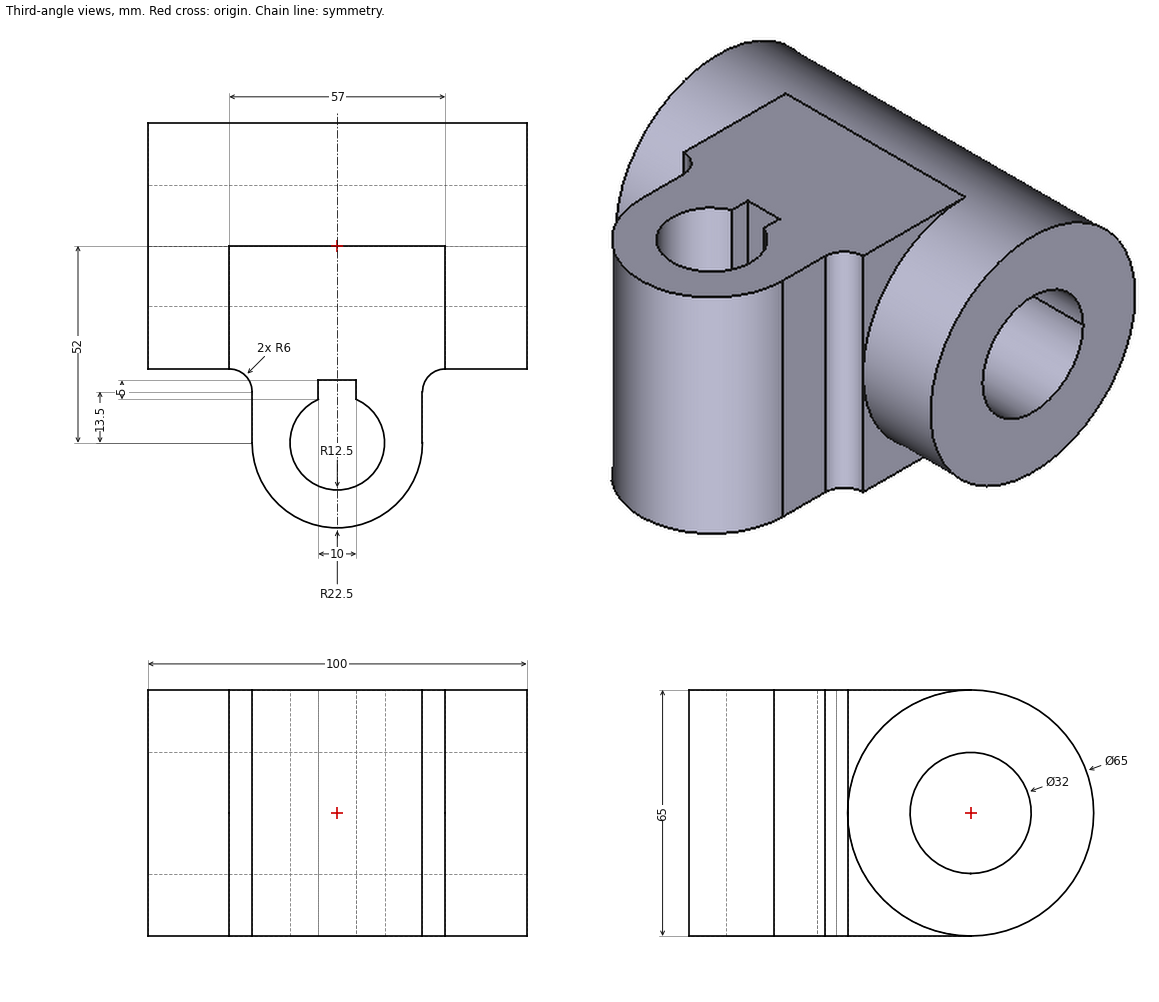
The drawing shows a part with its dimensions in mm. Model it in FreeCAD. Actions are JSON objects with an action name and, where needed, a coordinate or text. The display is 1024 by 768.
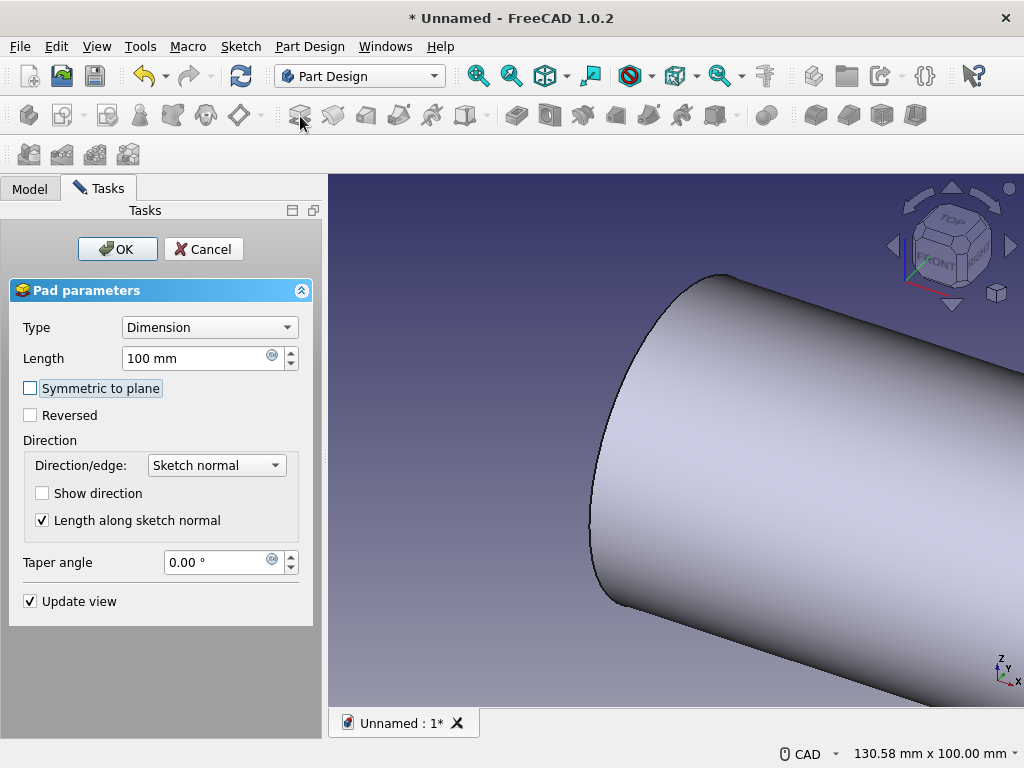
{"action": "left_click", "coordinate": [31, 388]}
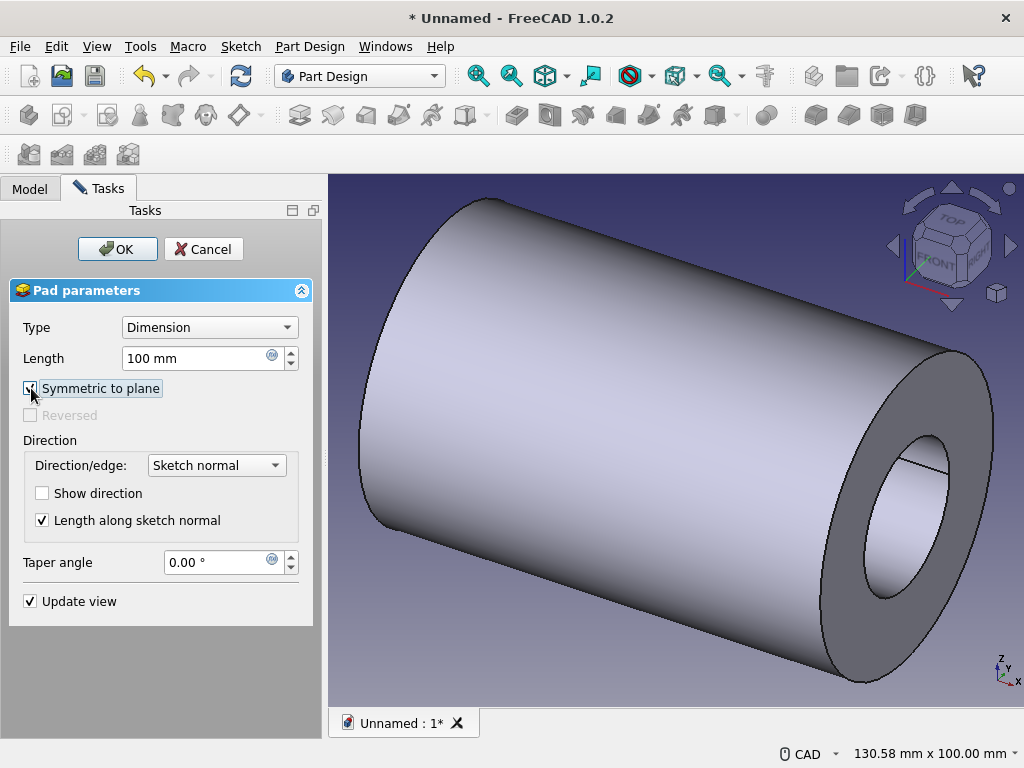
{"action": "left_click", "coordinate": [118, 249]}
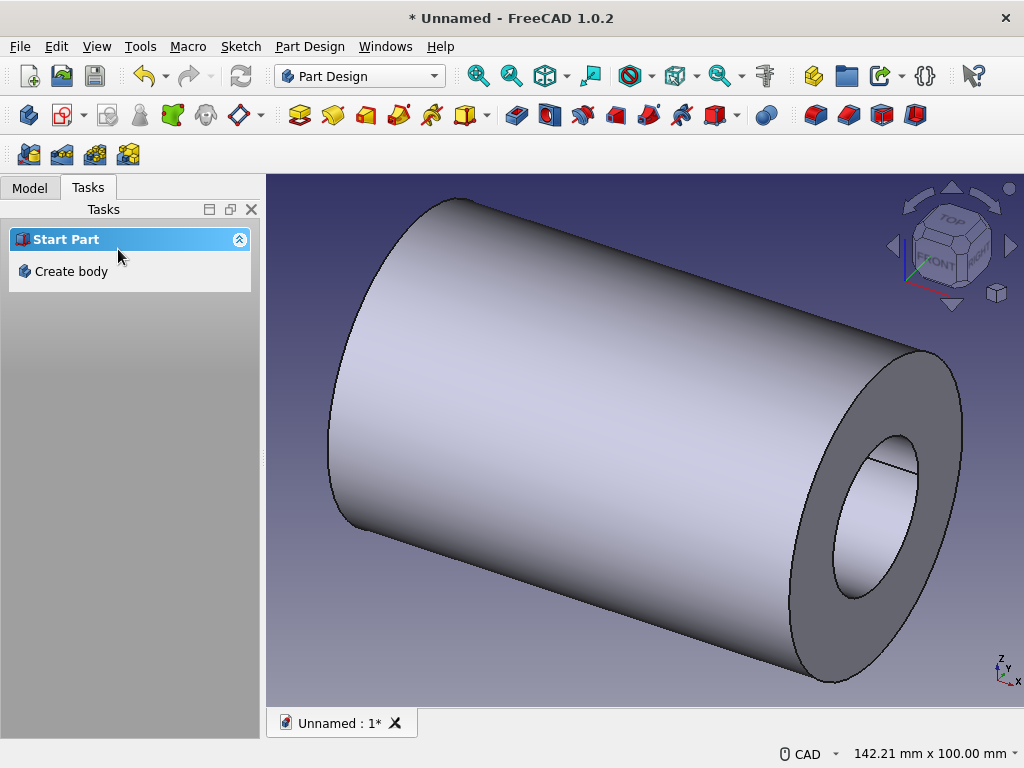
{"action": "key", "text": "v f"}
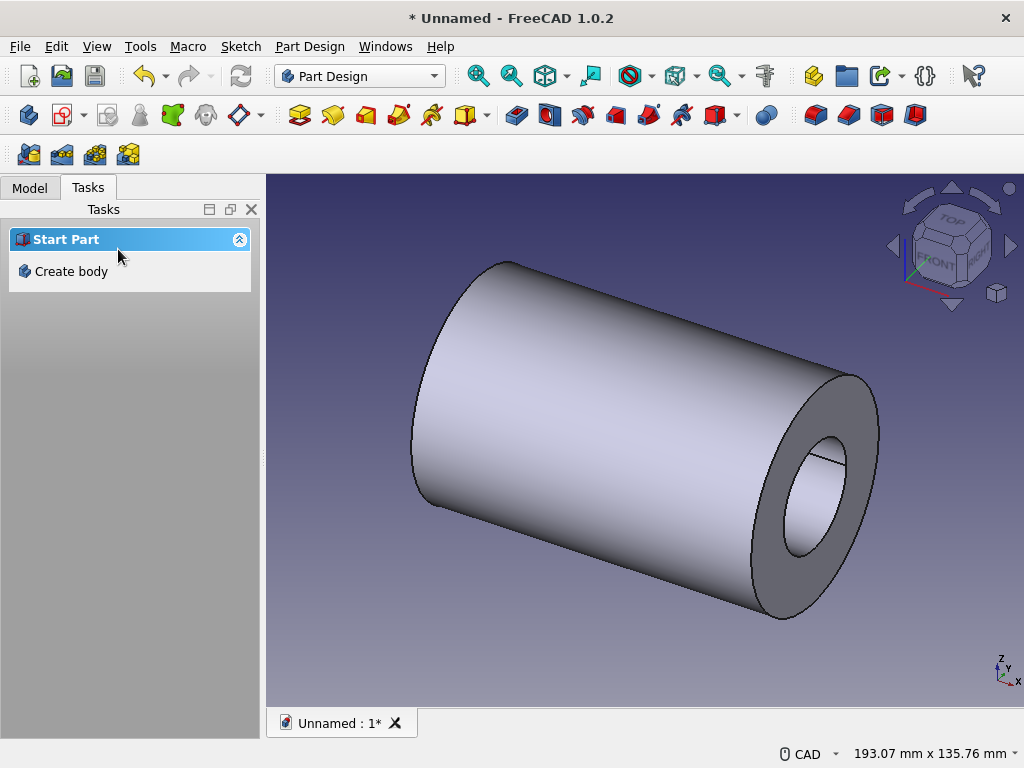
{"action": "left_click", "coordinate": [29, 116]}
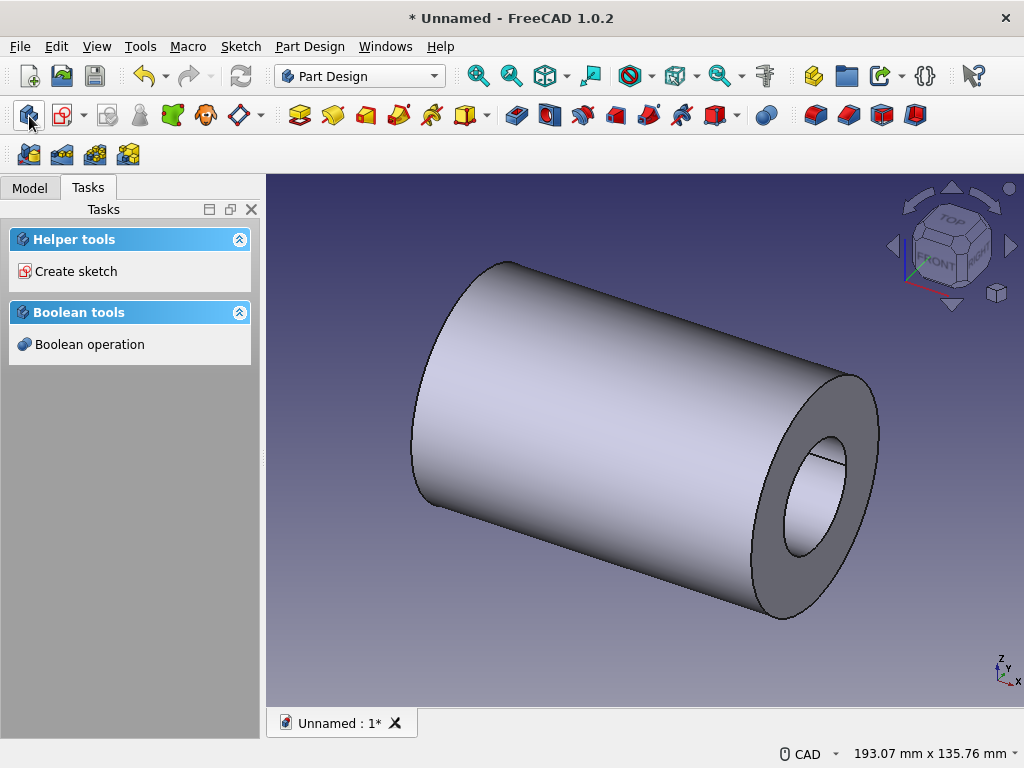
{"action": "left_click", "coordinate": [306, 667]}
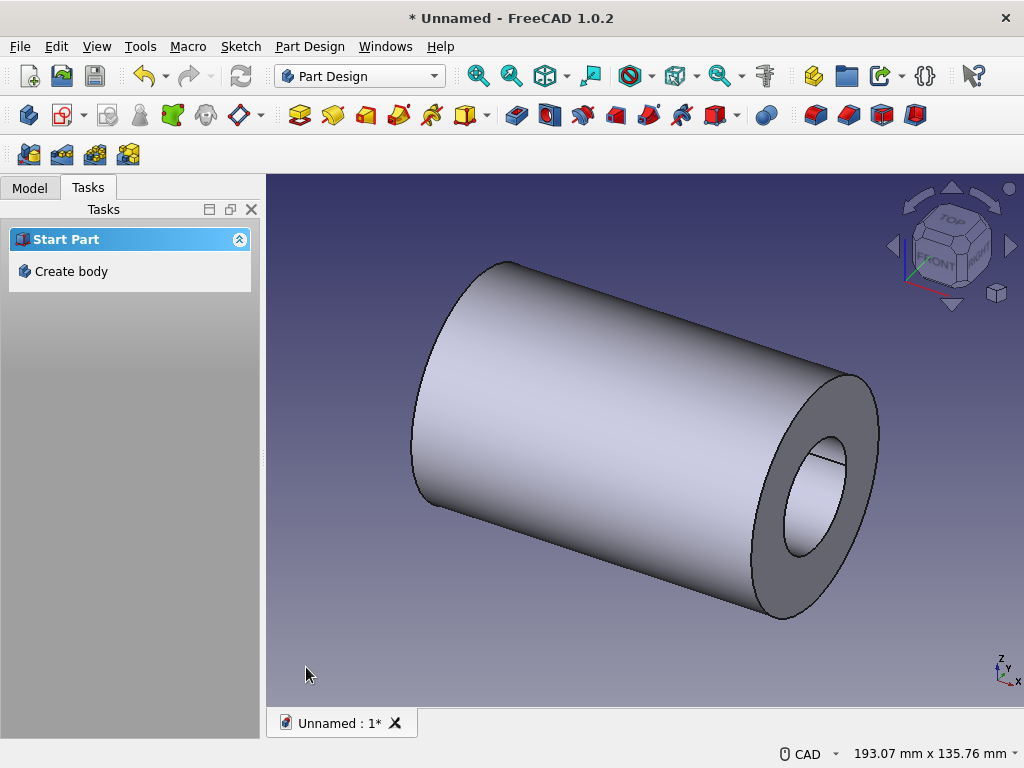
{"action": "left_click", "coordinate": [62, 116]}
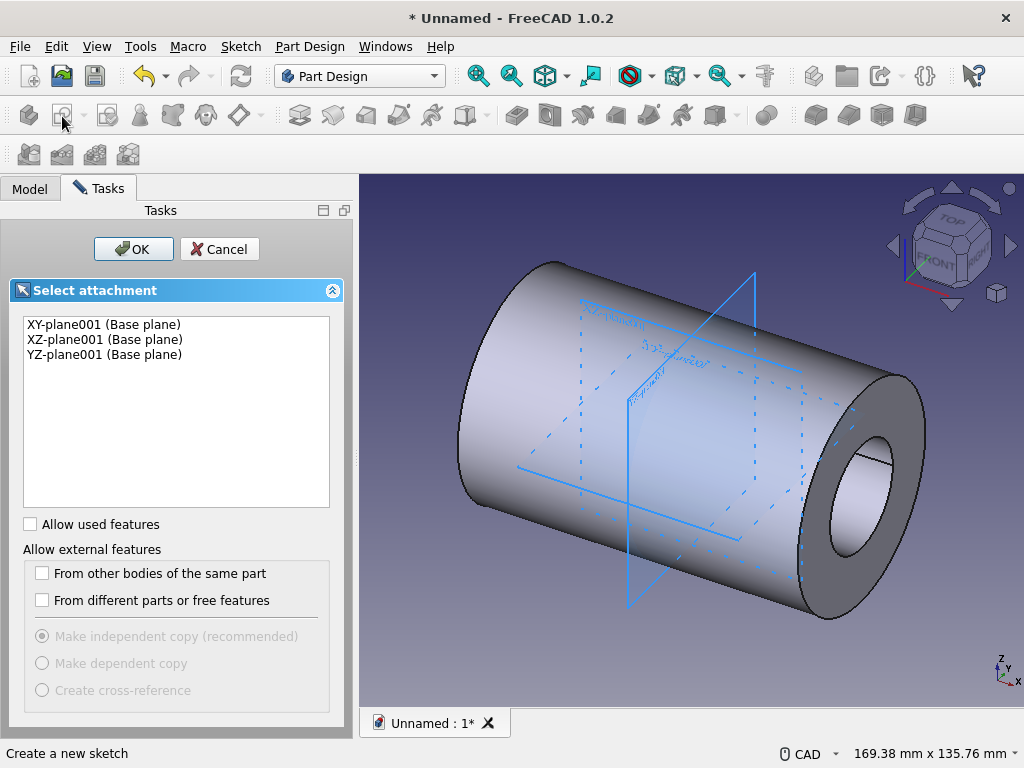
{"action": "left_click", "coordinate": [84, 324]}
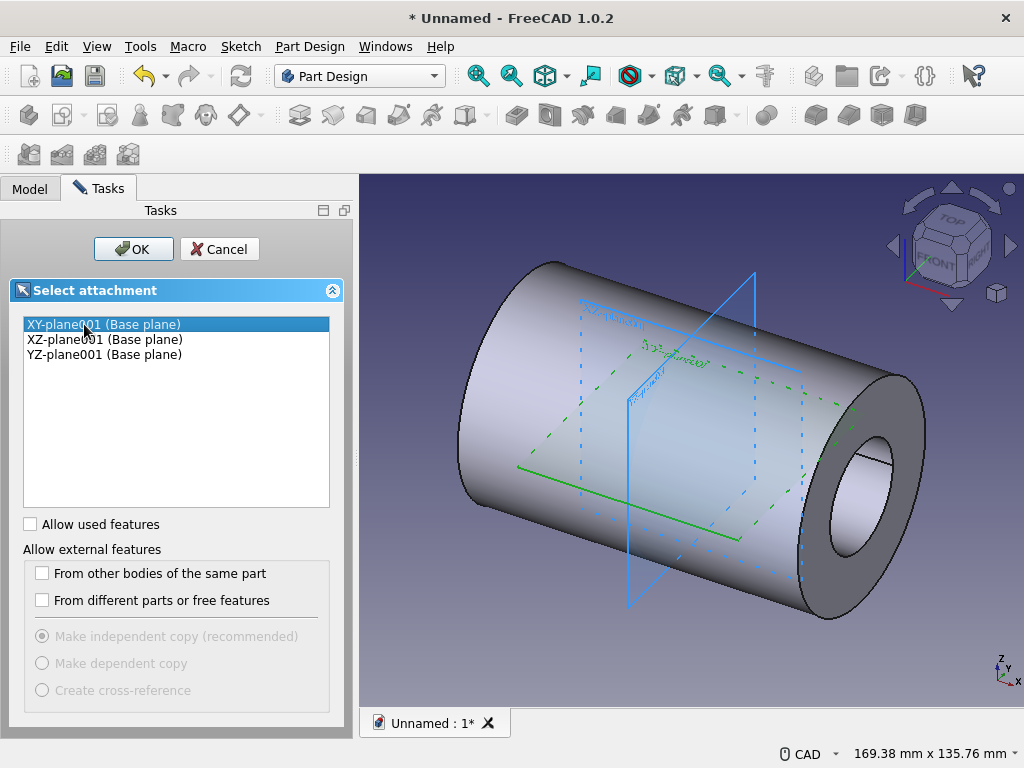
{"action": "left_click", "coordinate": [134, 249]}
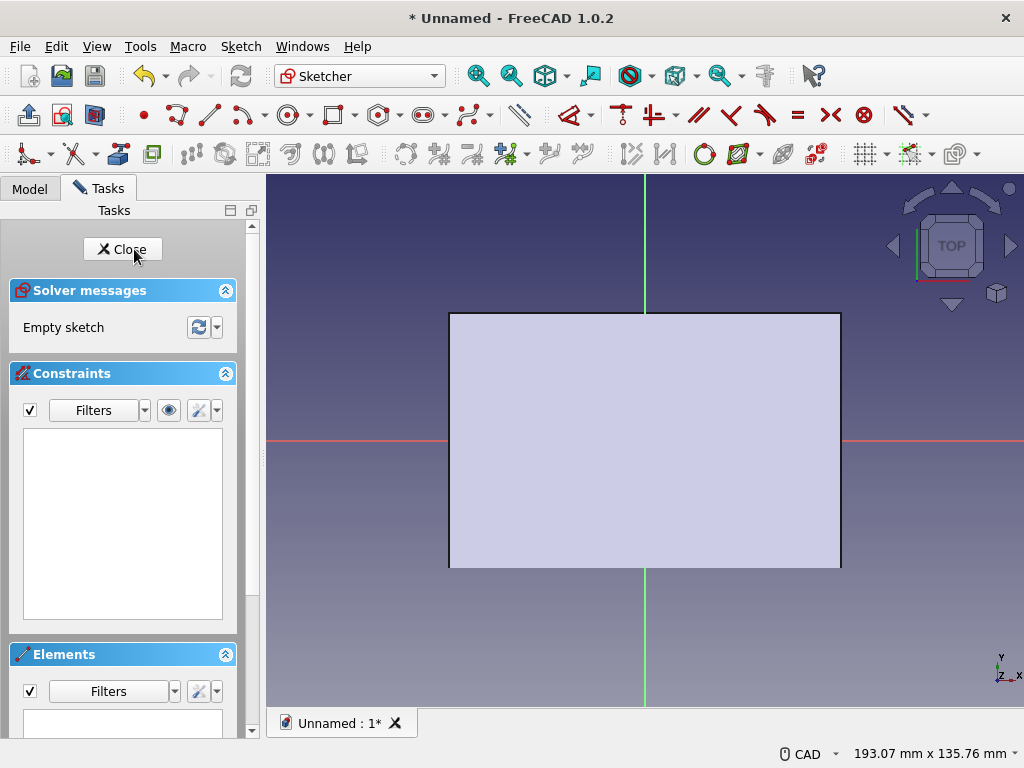
{"action": "scroll", "coordinate": [294, 202], "scroll_direction": "down", "scroll_amount": 1}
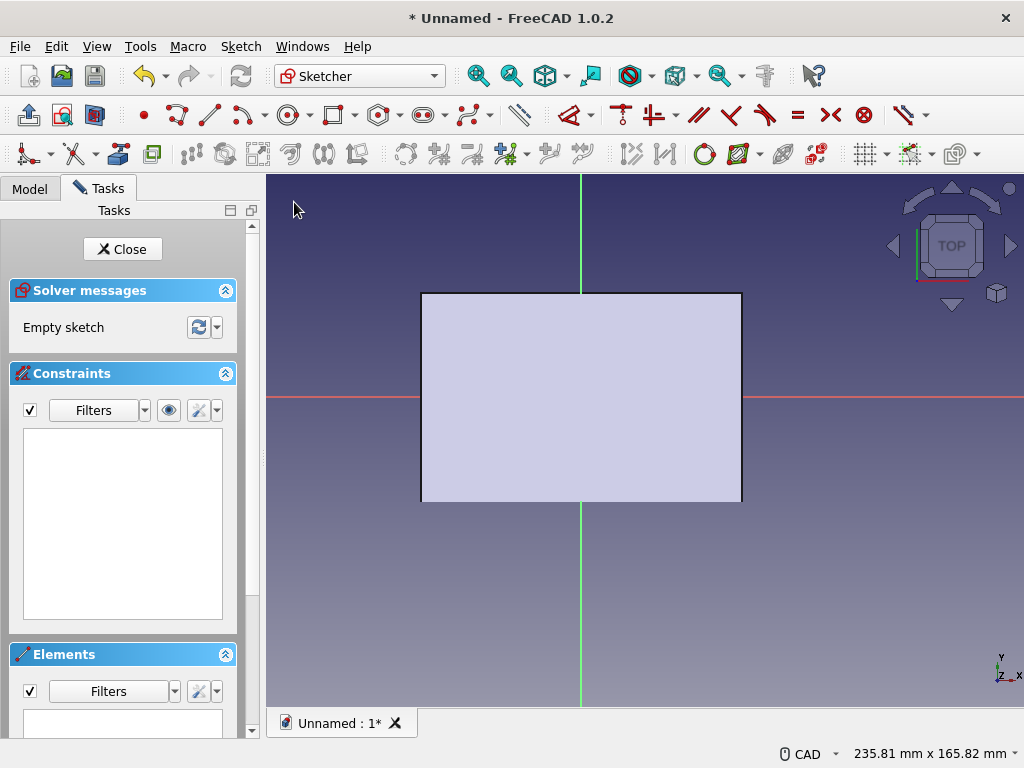
{"action": "scroll", "coordinate": [591, 673], "scroll_direction": "up", "scroll_amount": 2}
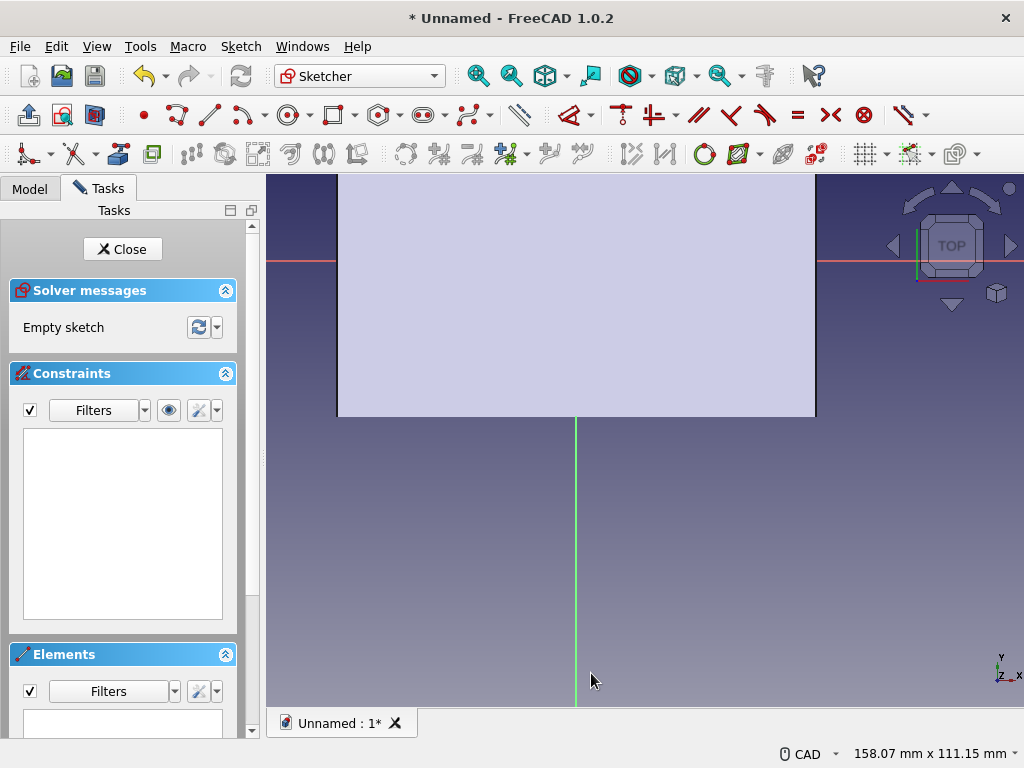
{"action": "left_click", "coordinate": [210, 116]}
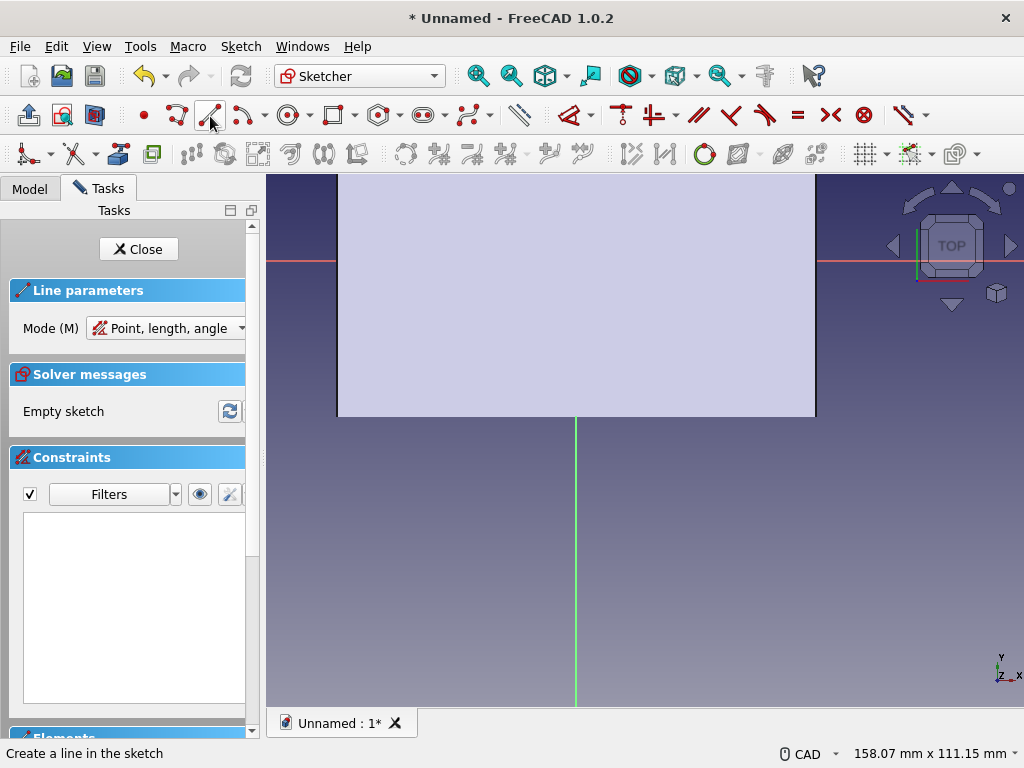
{"action": "left_click", "coordinate": [469, 446]}
{"action": "left_click", "coordinate": [469, 511]}